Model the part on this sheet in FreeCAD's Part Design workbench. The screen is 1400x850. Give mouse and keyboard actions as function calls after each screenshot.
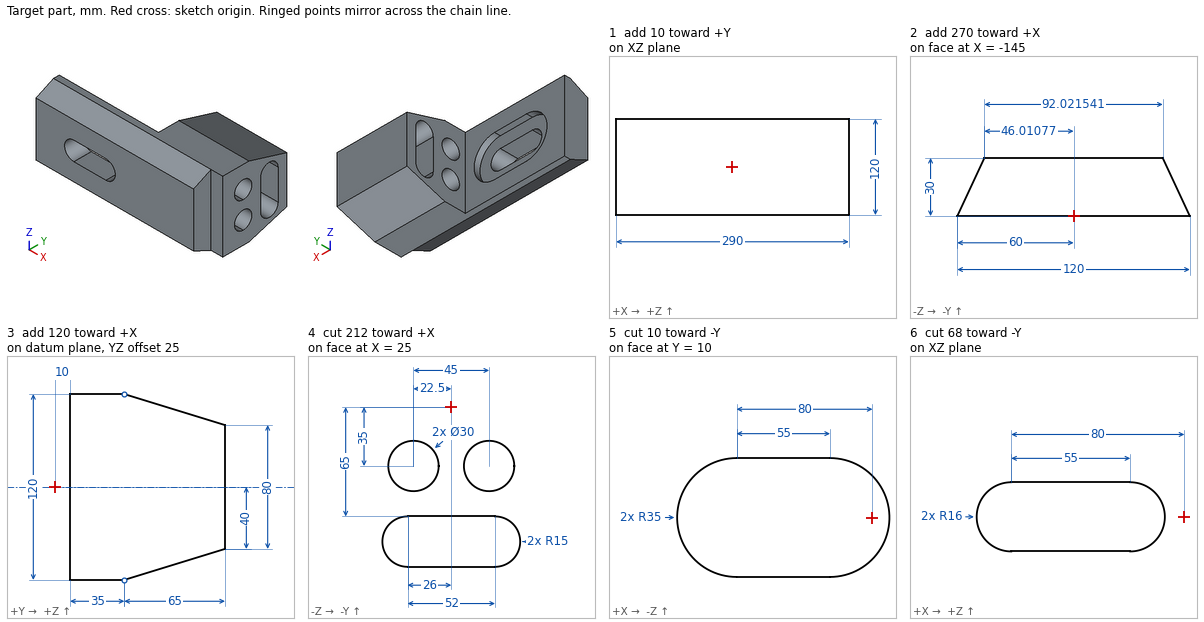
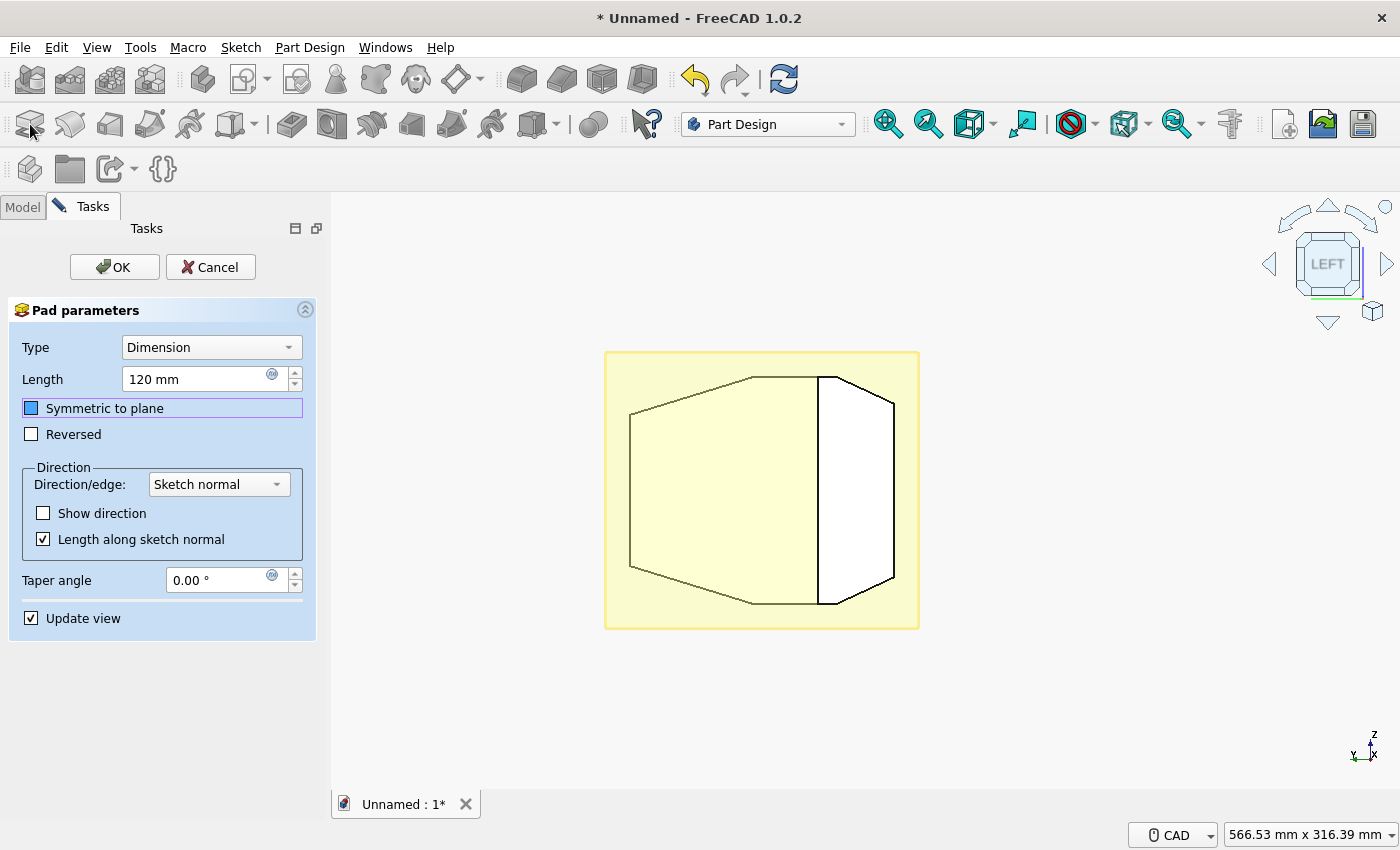
click(115, 267)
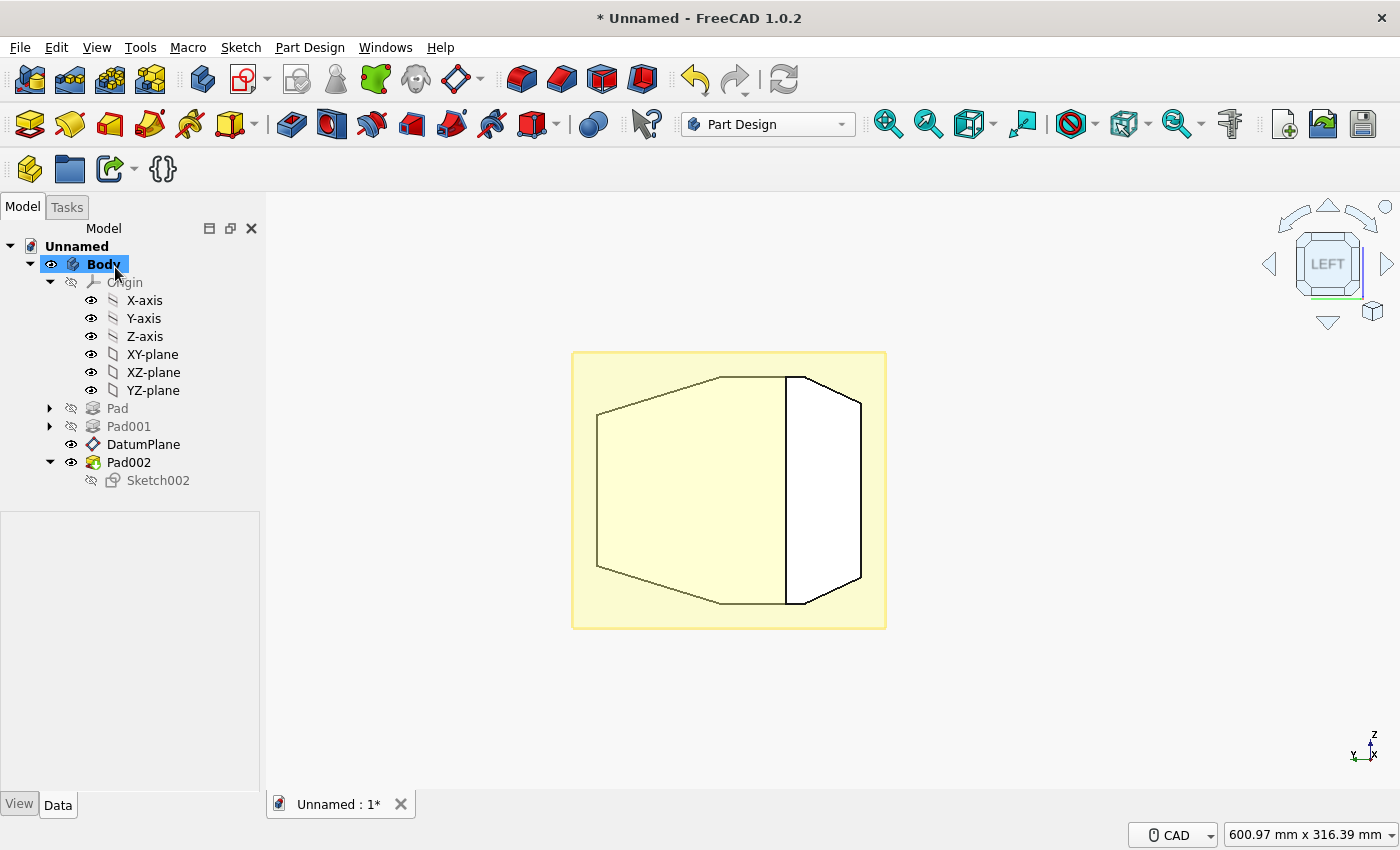
click(116, 444)
key(space)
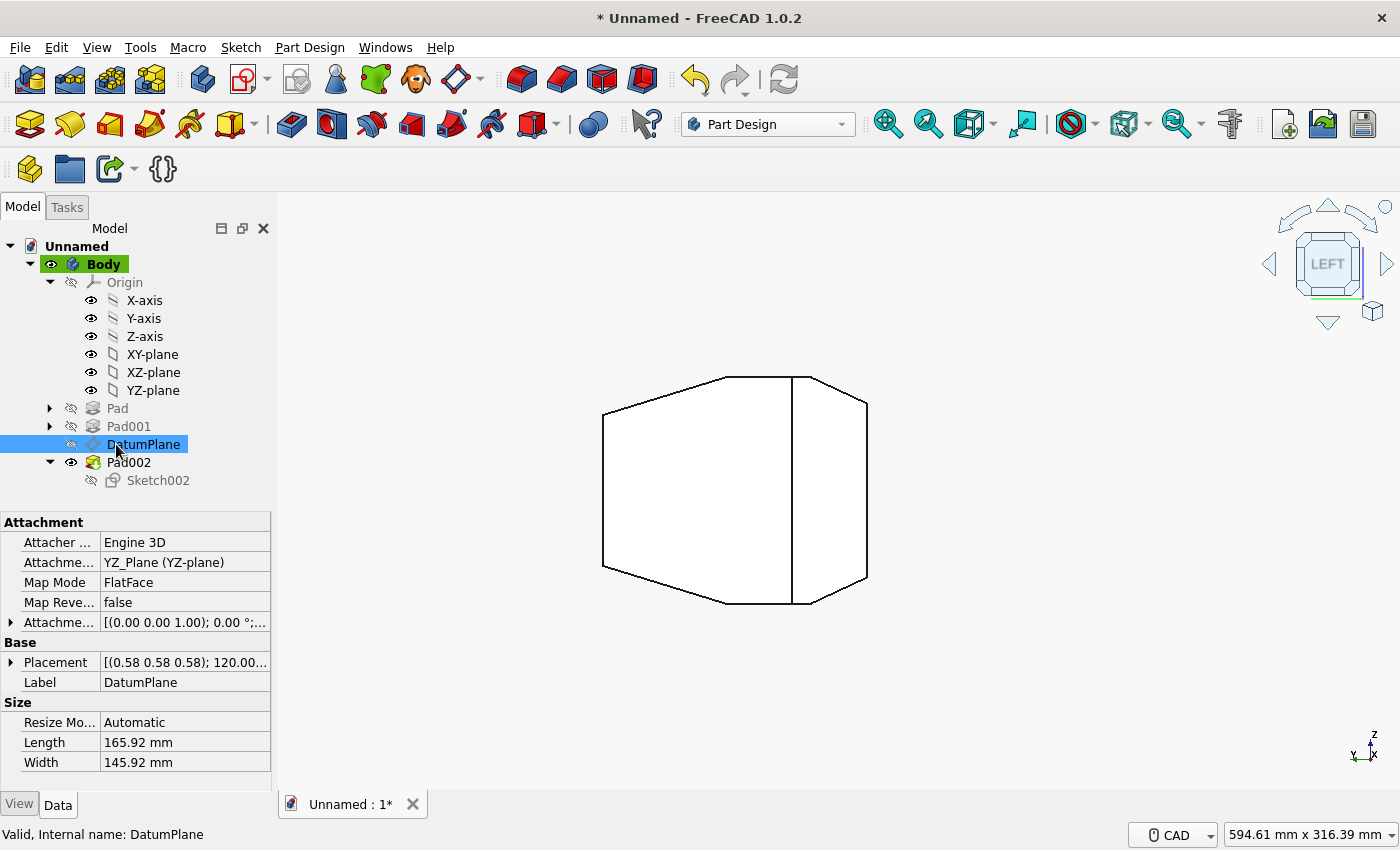
click(890, 124)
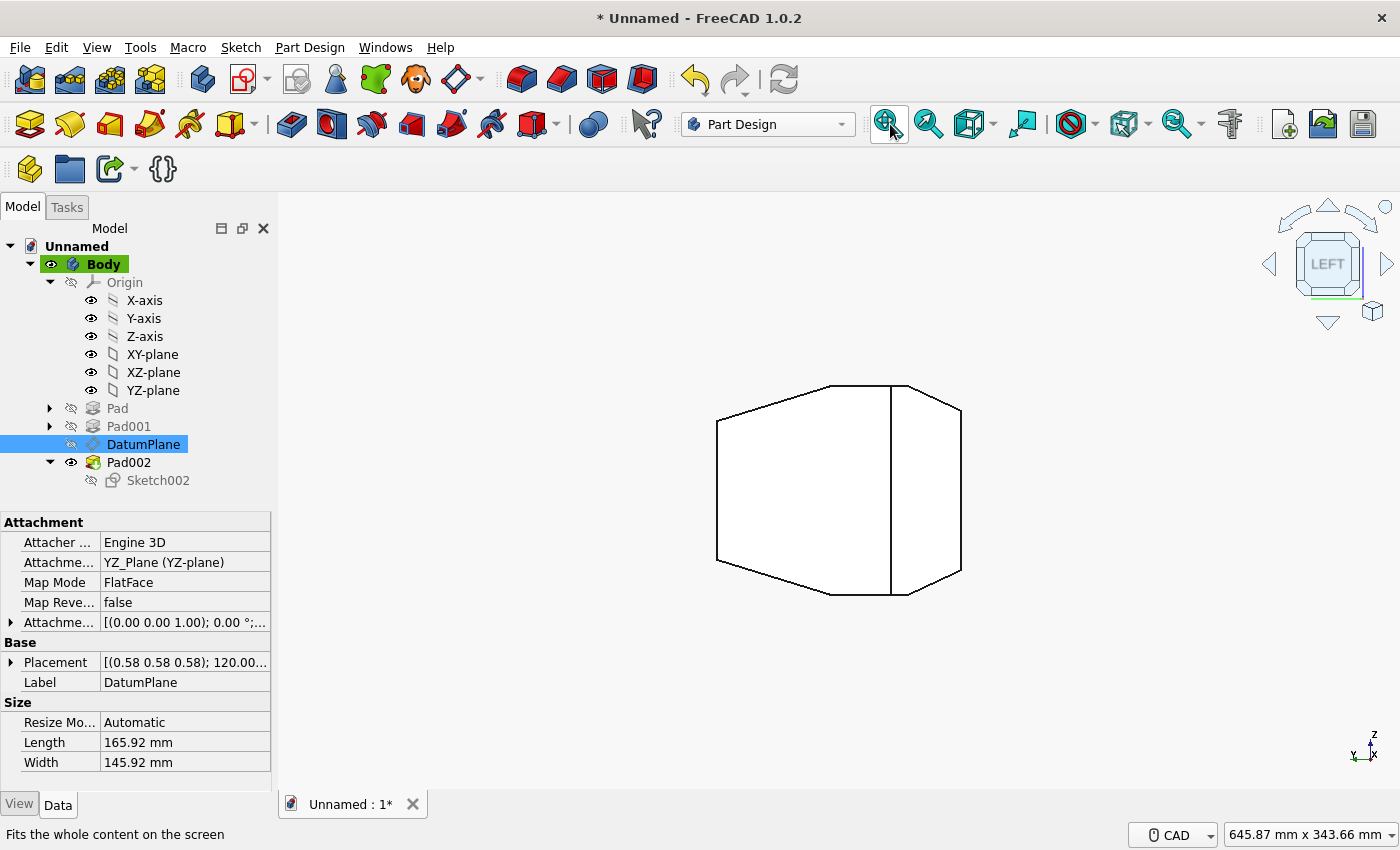
click(804, 489)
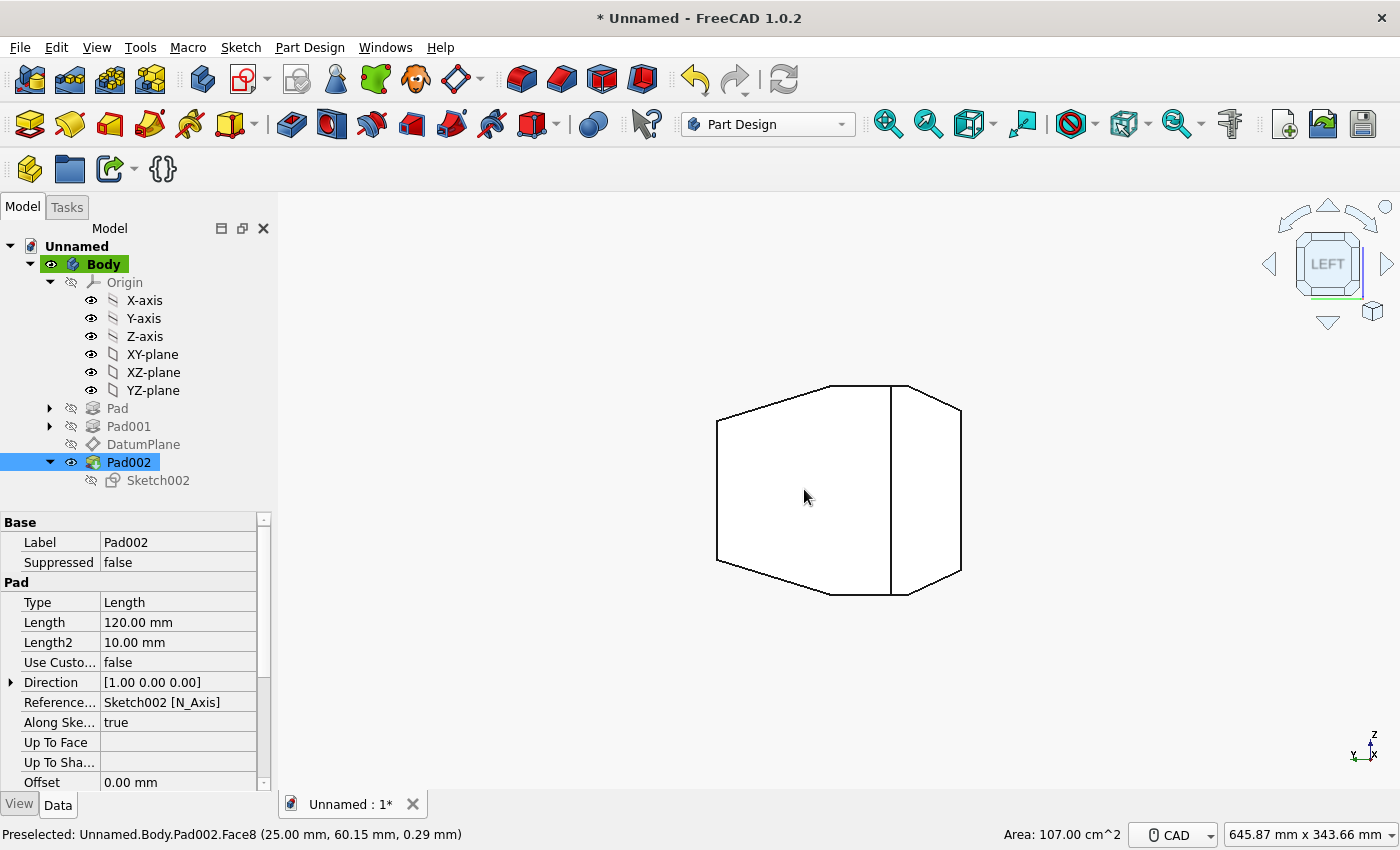
click(244, 80)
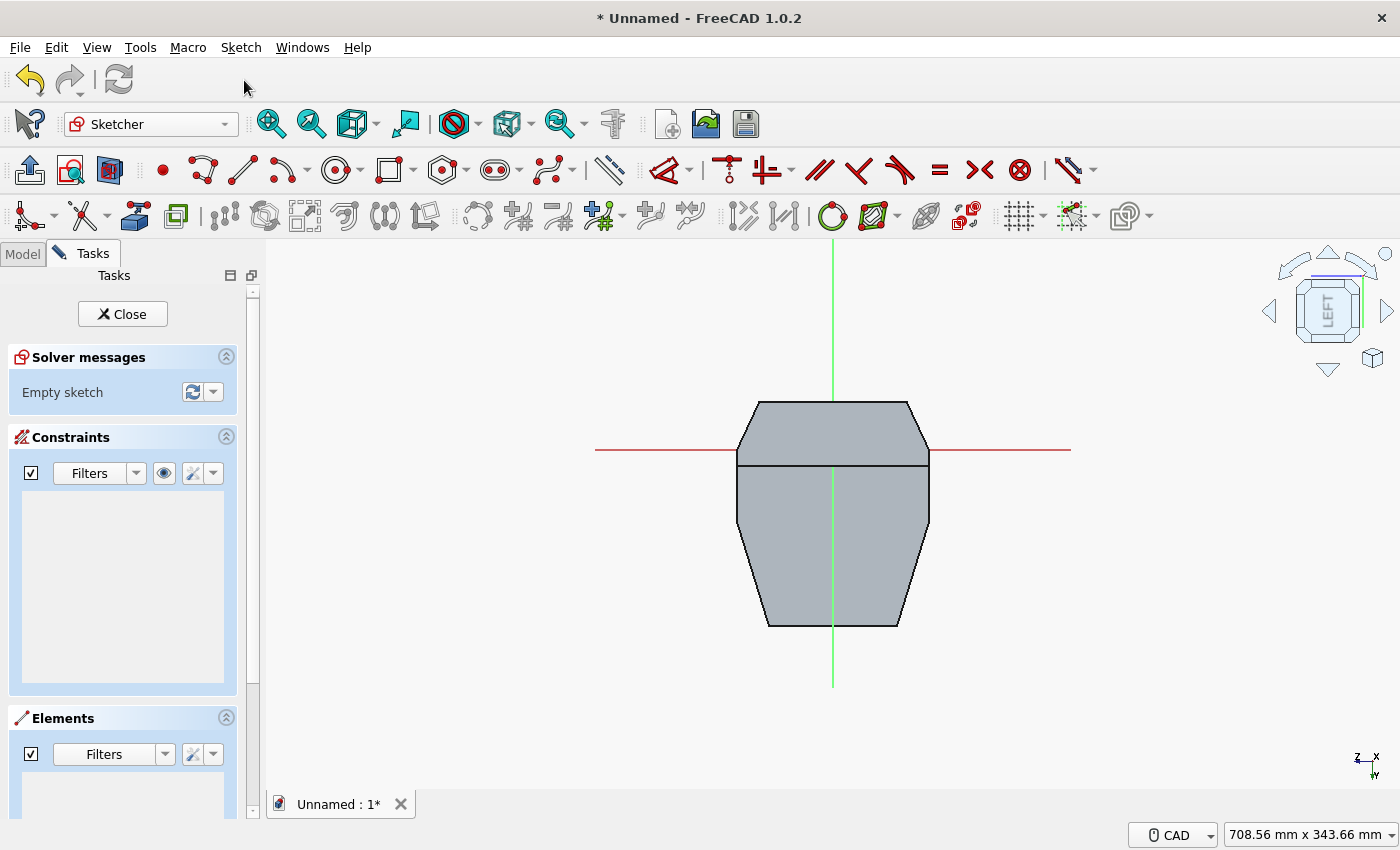
scroll(889, 536, up, 4)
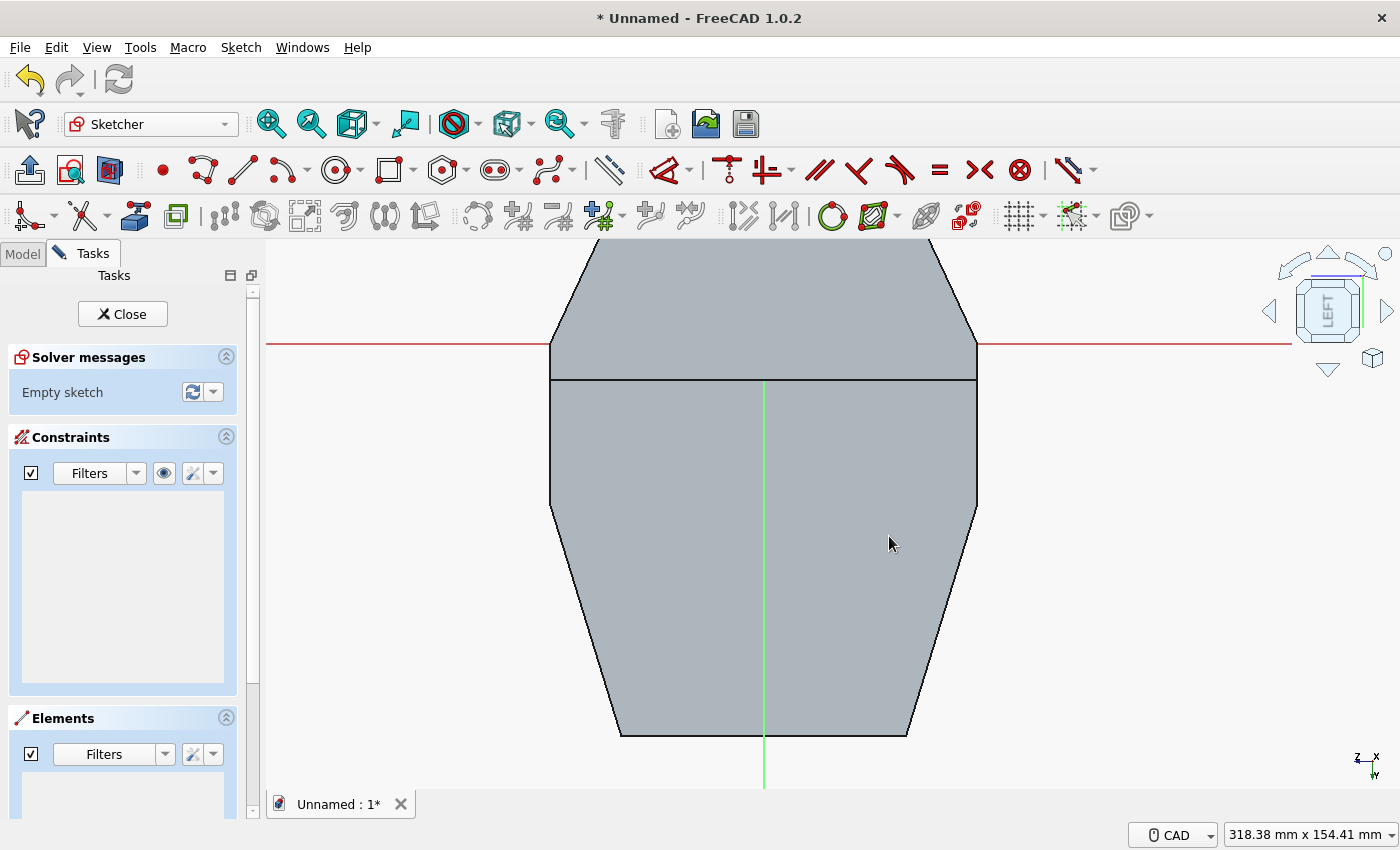
key(g)
key(s)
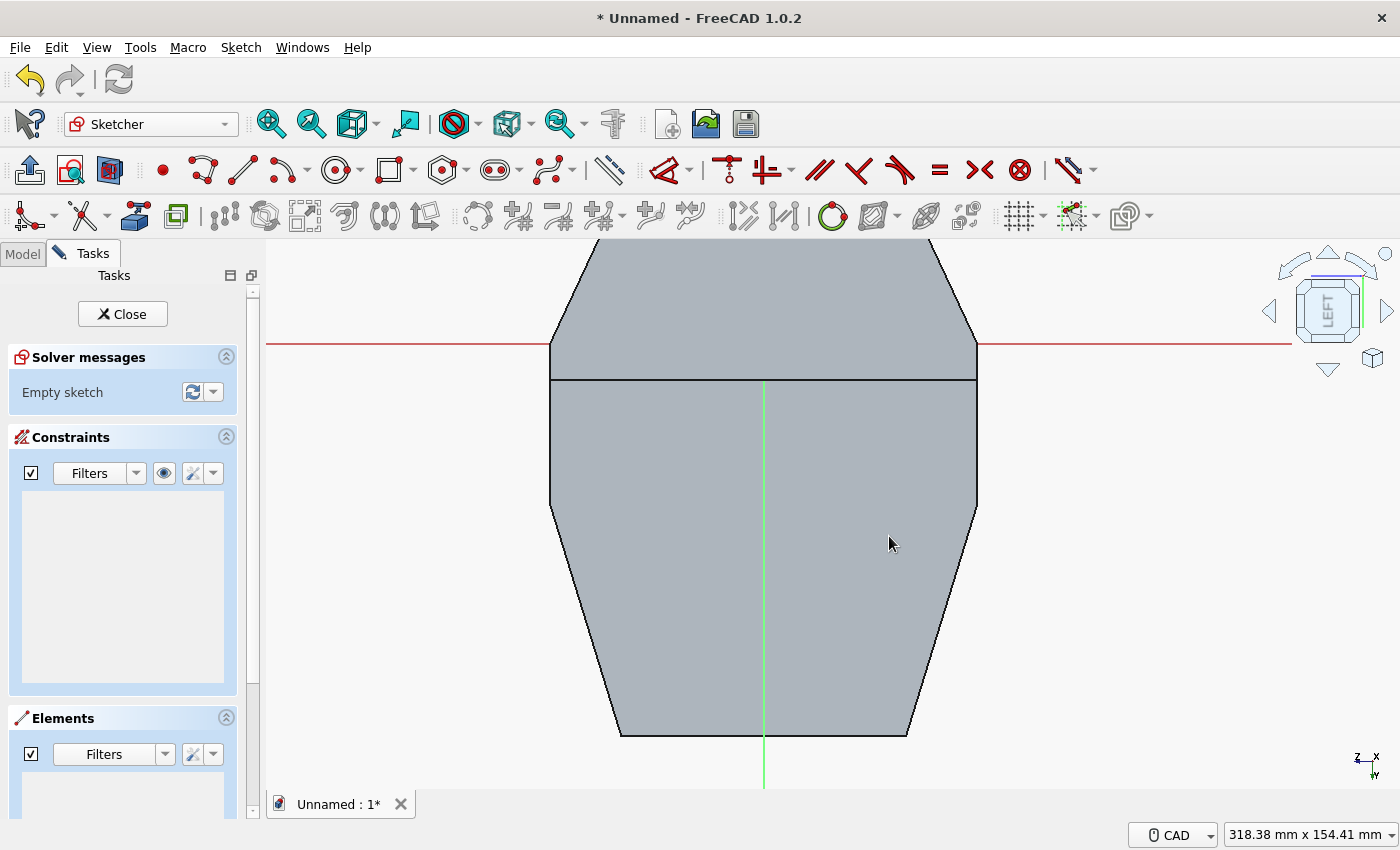
click(671, 629)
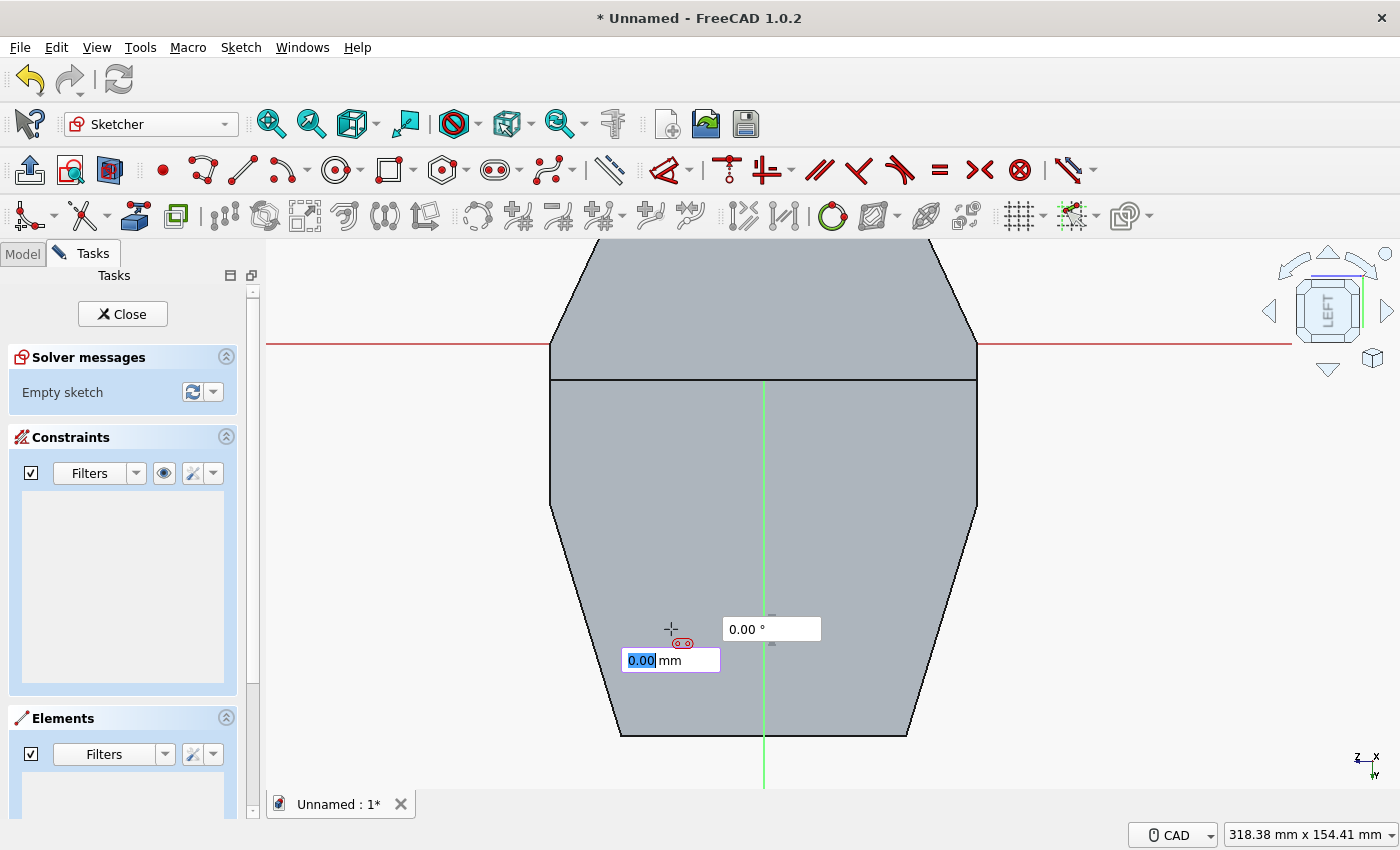
click(856, 629)